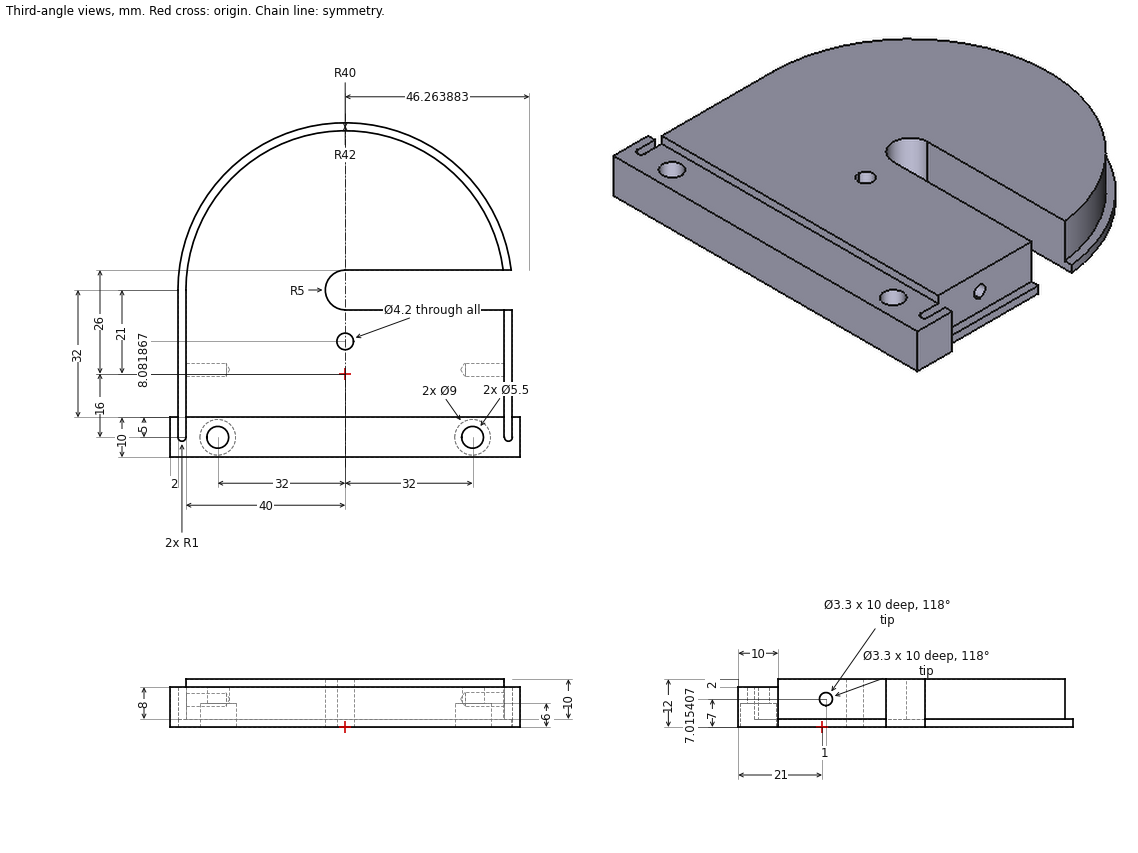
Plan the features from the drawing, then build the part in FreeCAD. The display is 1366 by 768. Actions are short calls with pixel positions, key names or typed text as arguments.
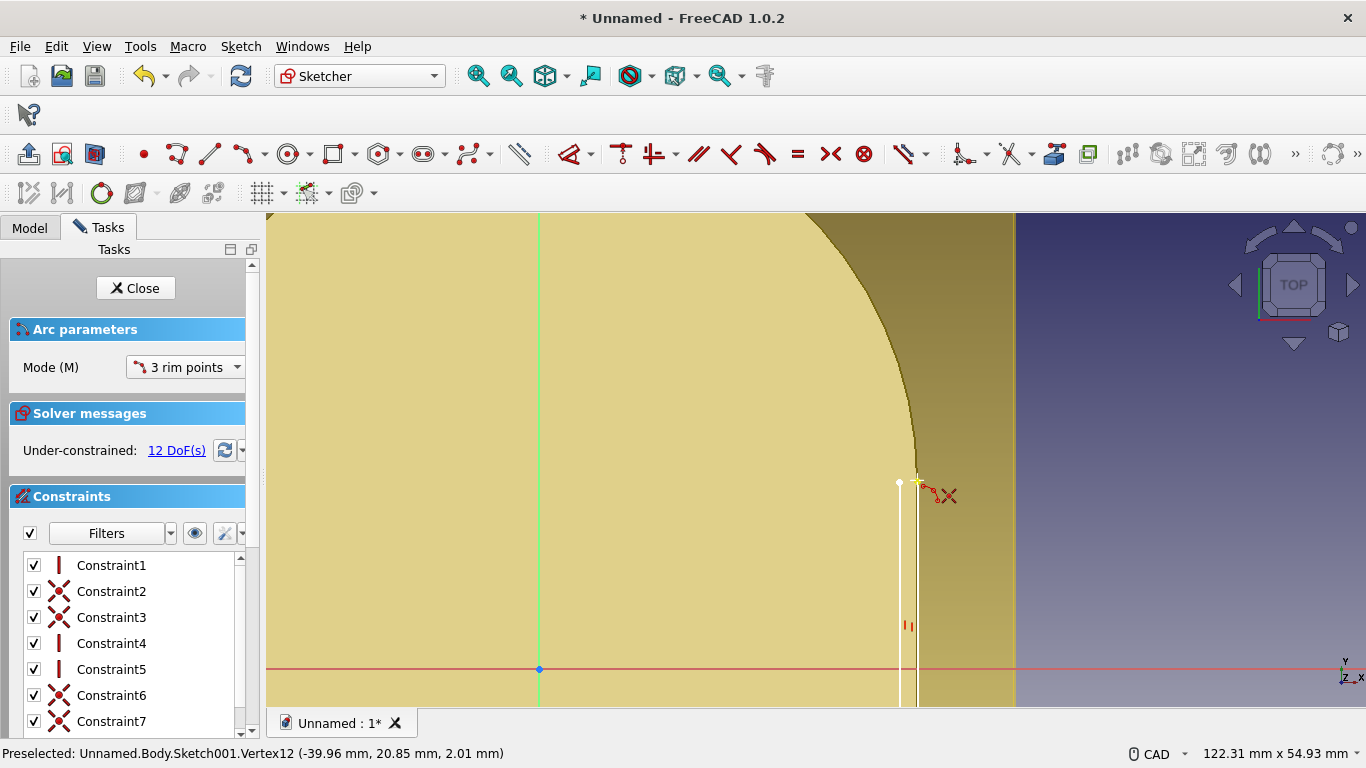
click(918, 481)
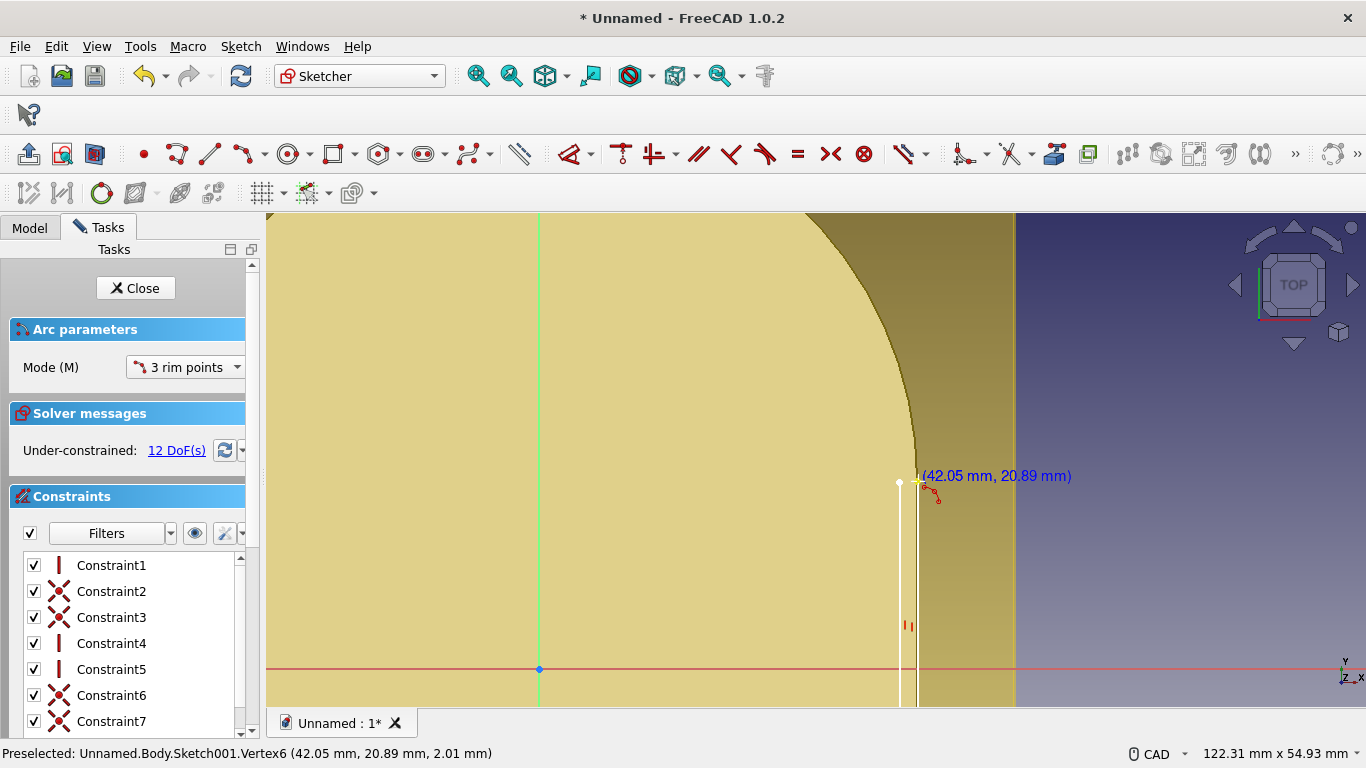
scroll(917, 480, down, 4)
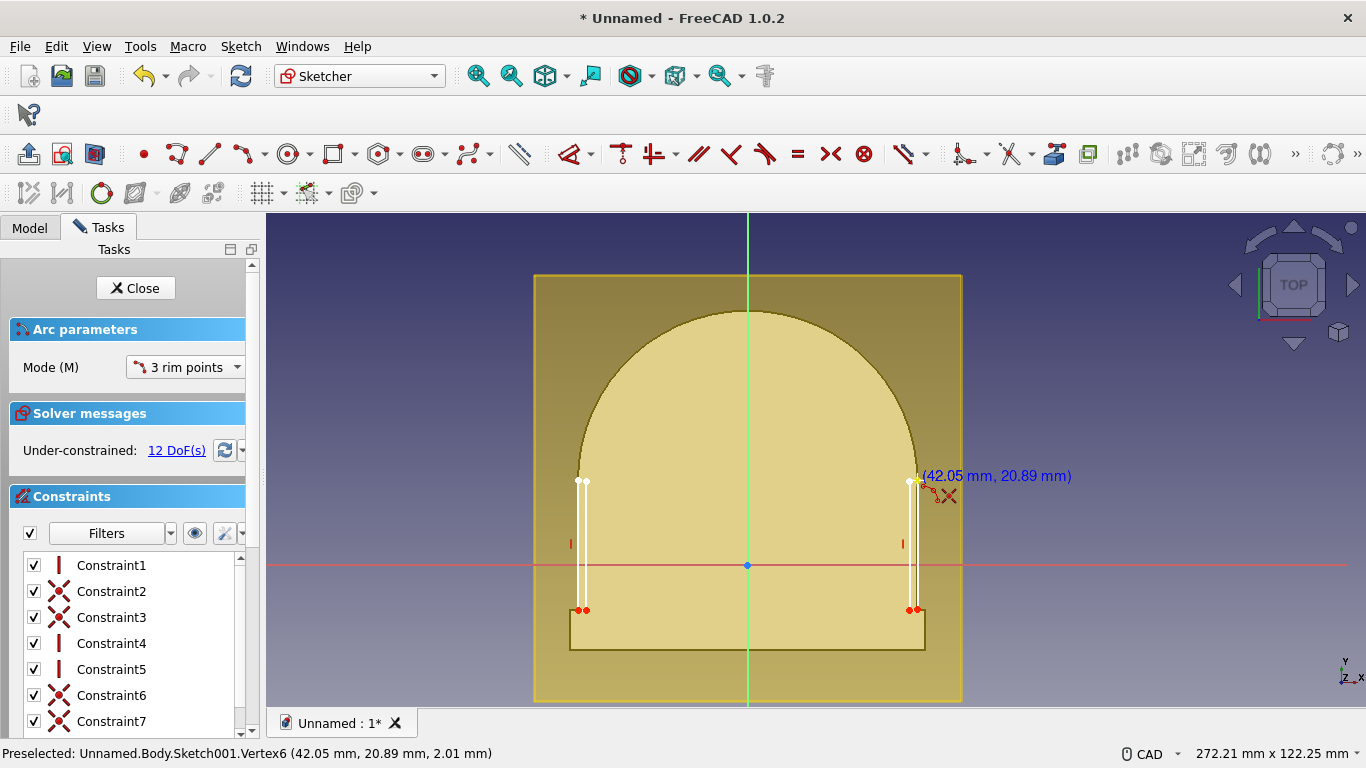
scroll(578, 480, up, 4)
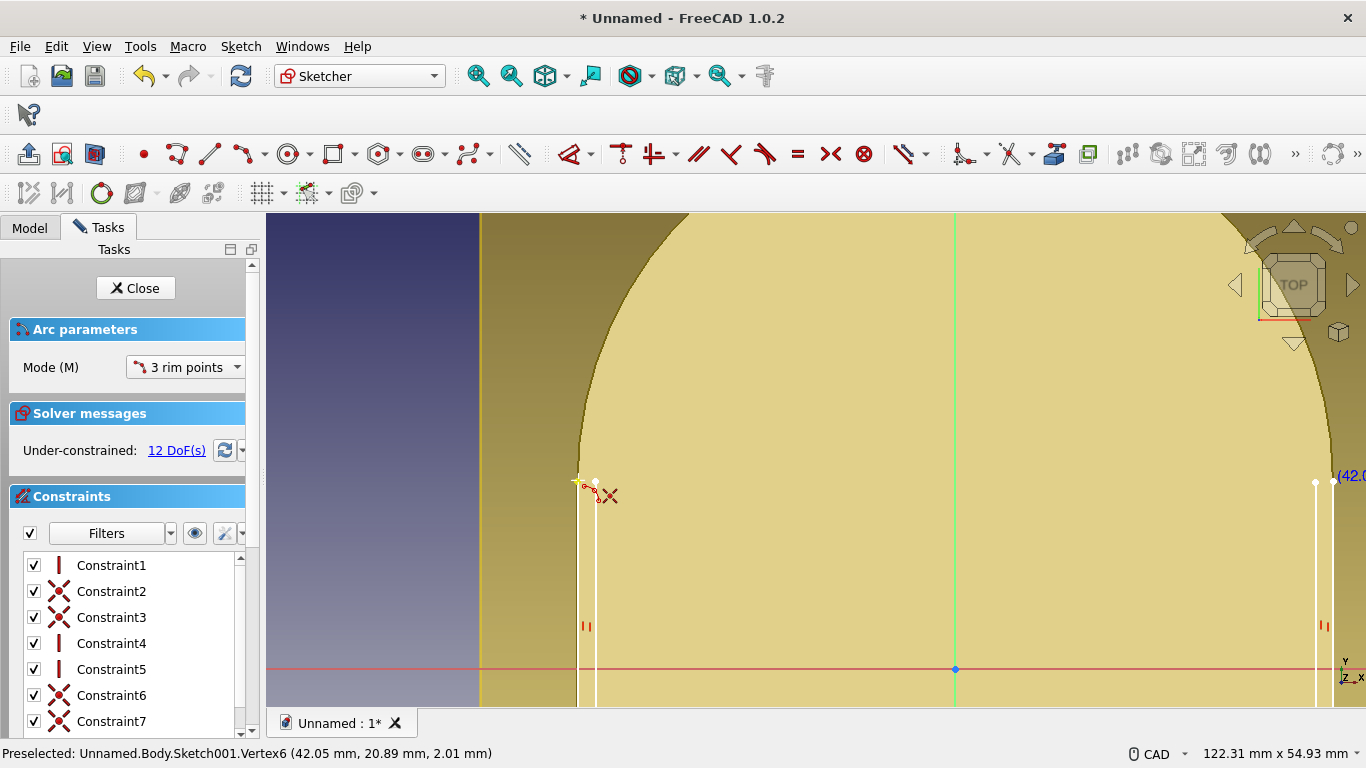
click(578, 482)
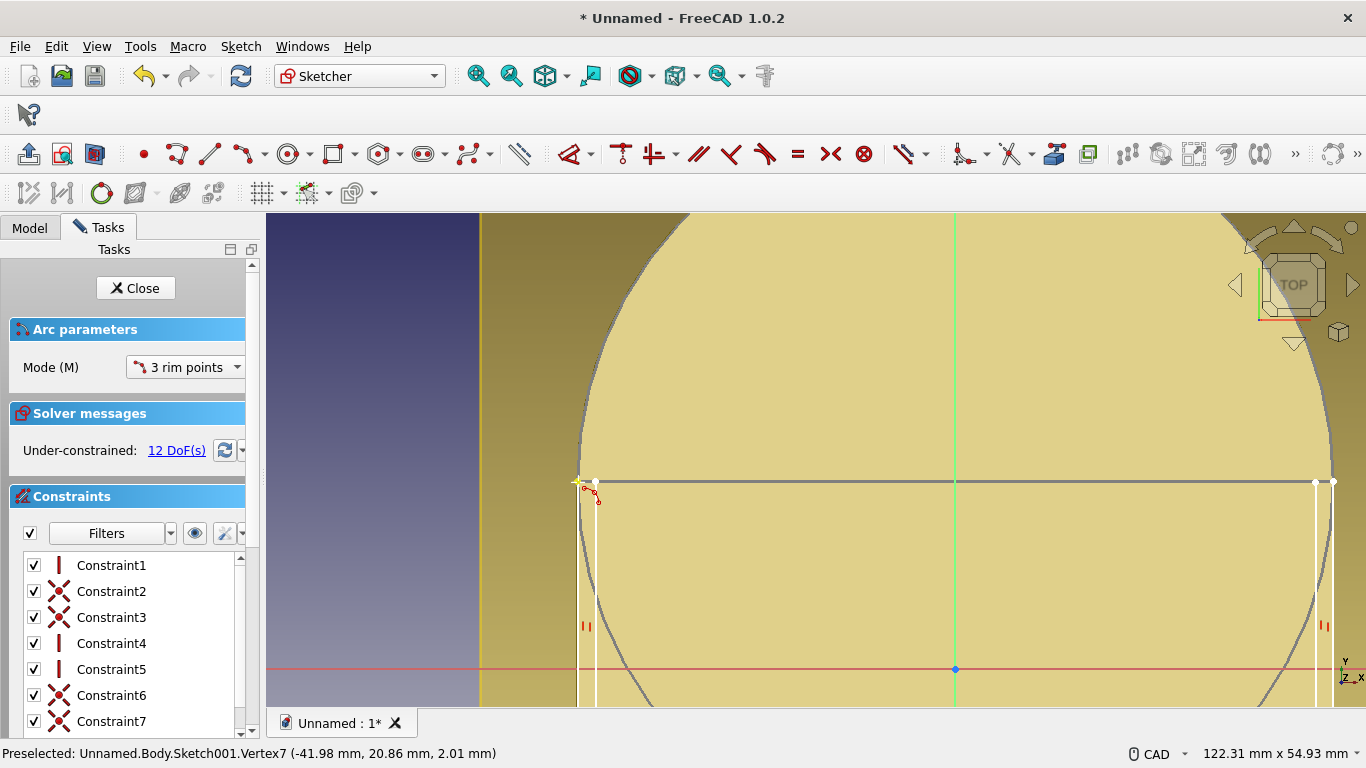
scroll(578, 480, down, 4)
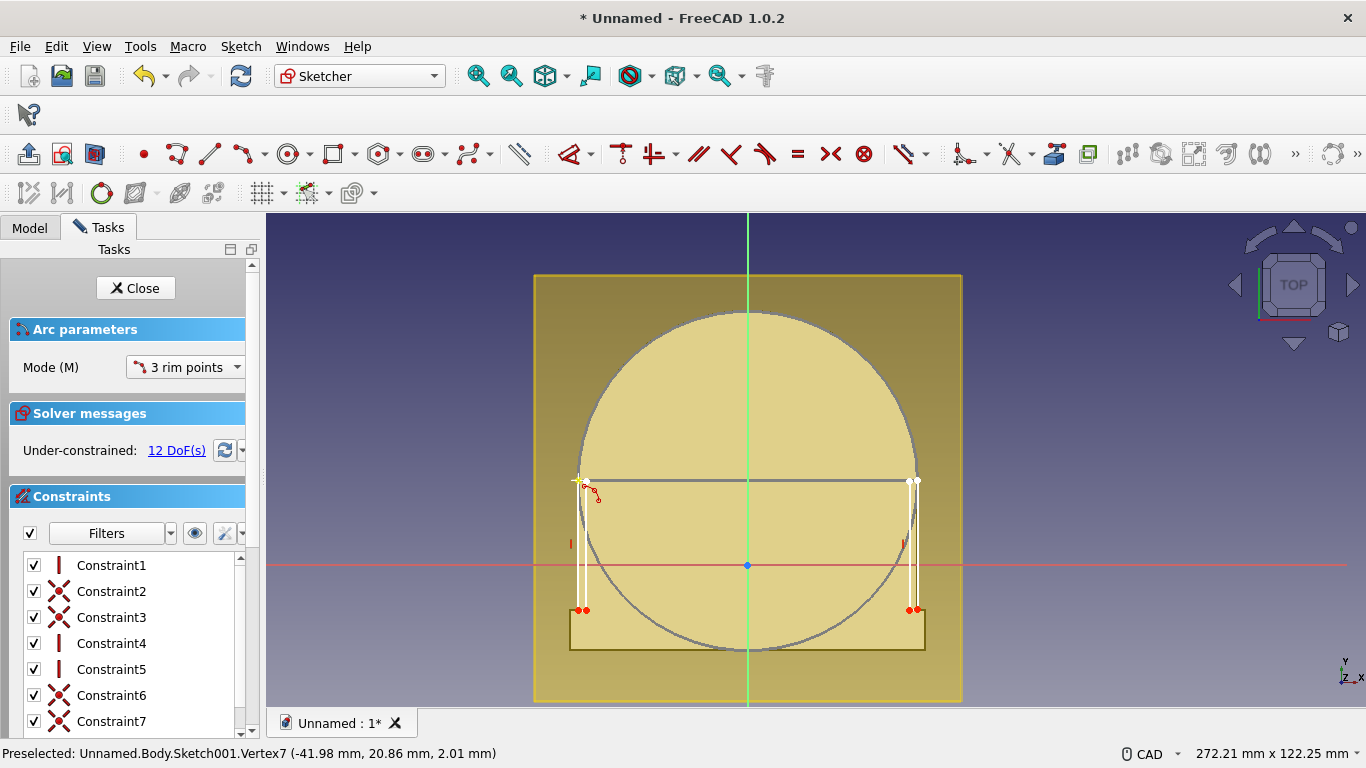
click(800, 319)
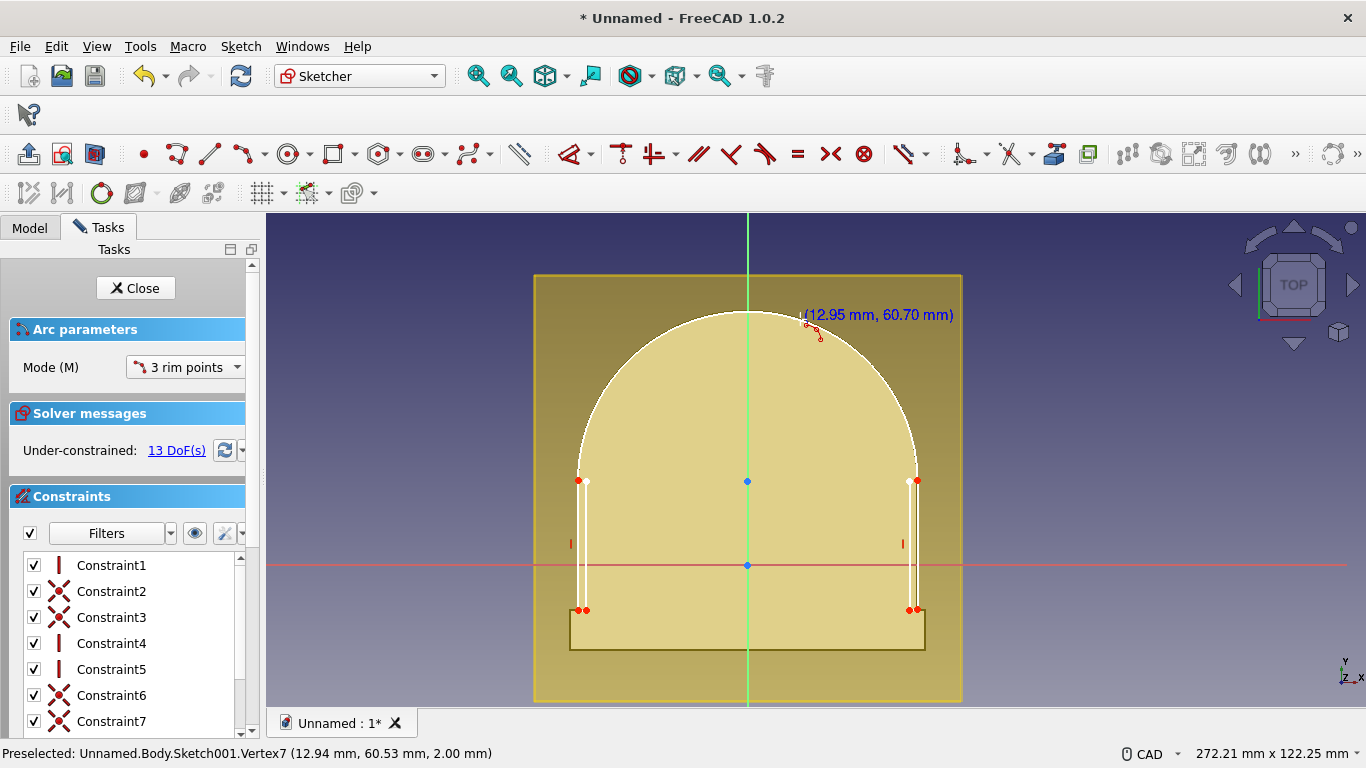
scroll(586, 480, up, 4)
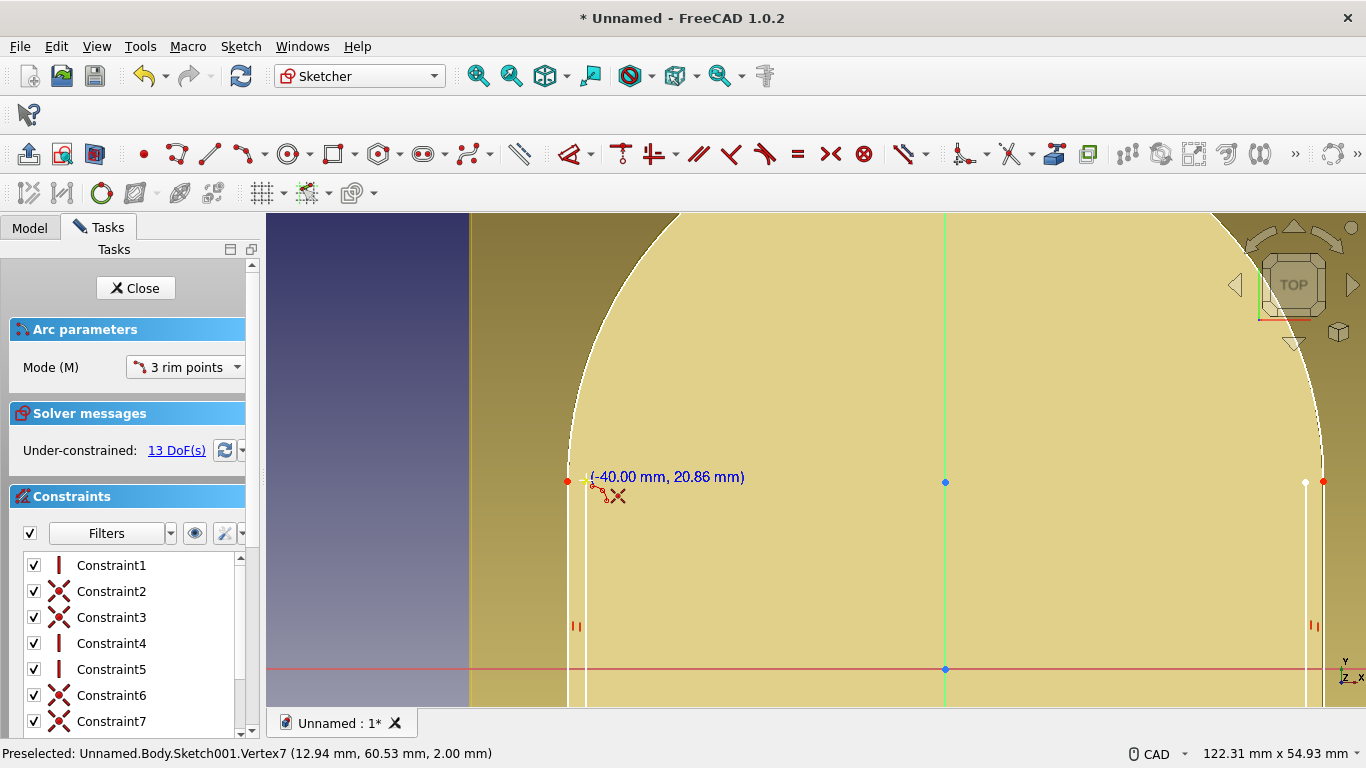
click(586, 482)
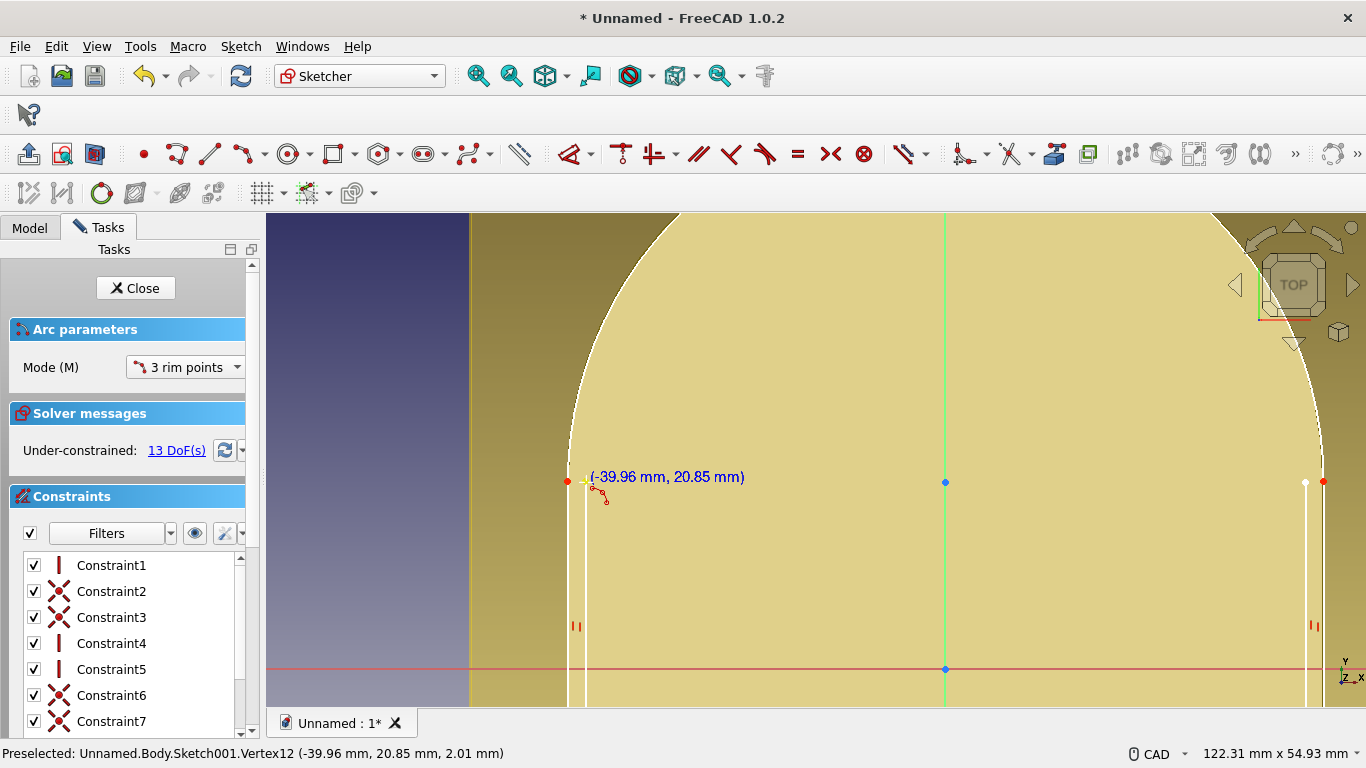
scroll(586, 480, down, 4)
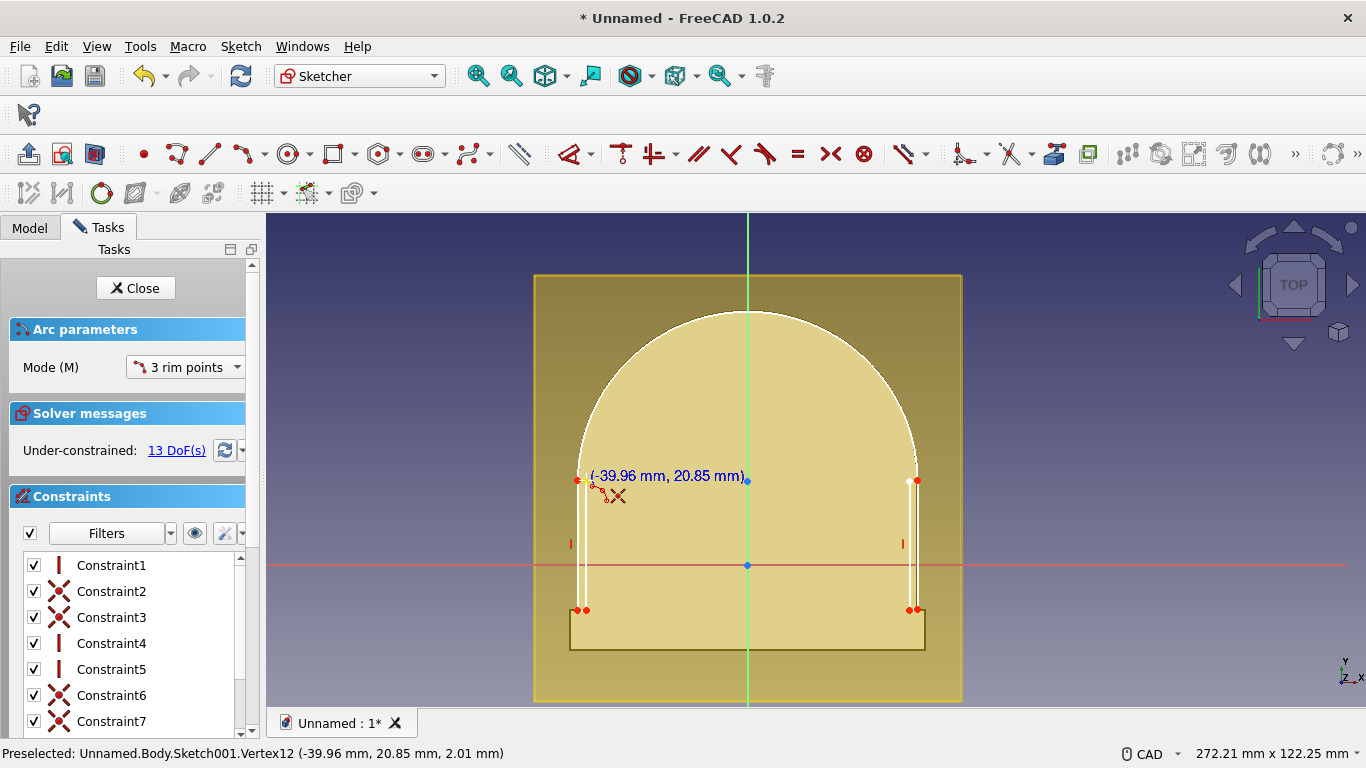
scroll(909, 480, up, 4)